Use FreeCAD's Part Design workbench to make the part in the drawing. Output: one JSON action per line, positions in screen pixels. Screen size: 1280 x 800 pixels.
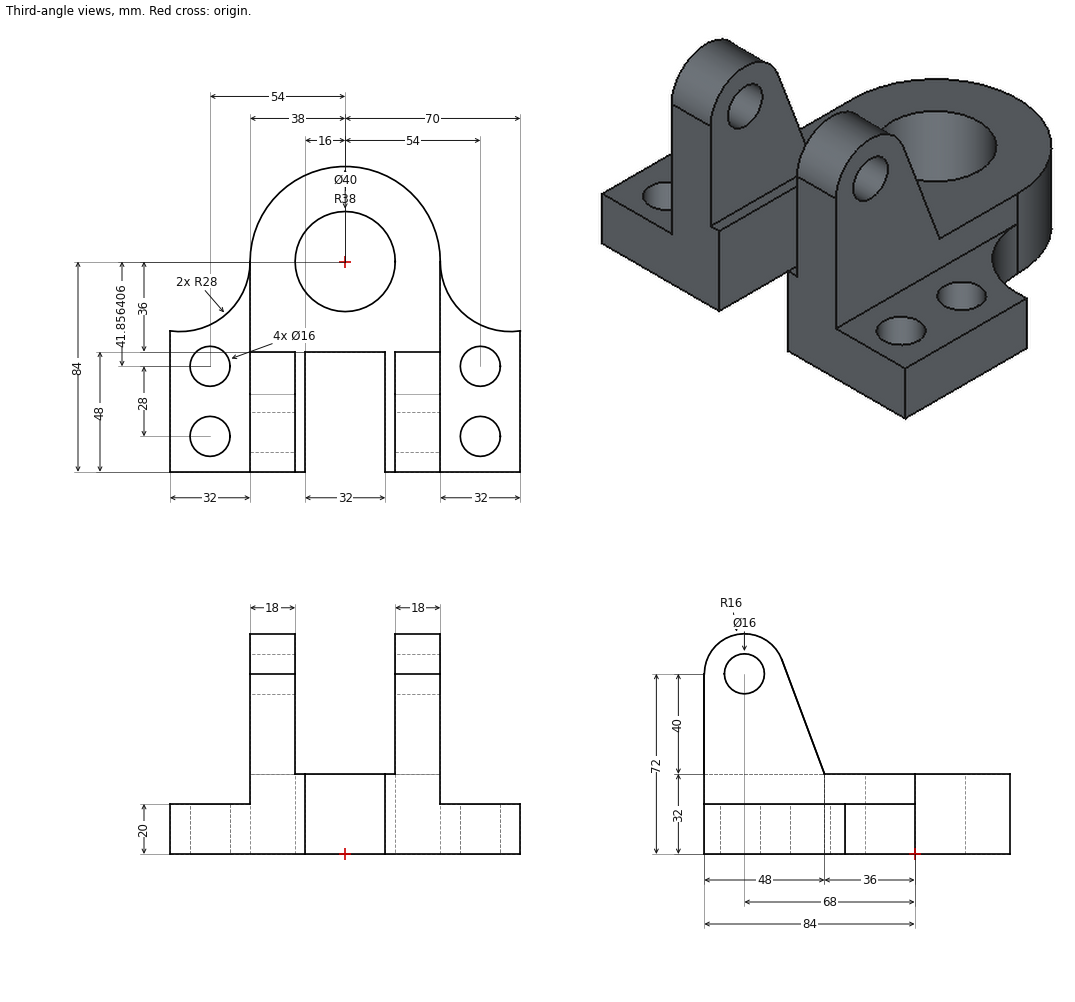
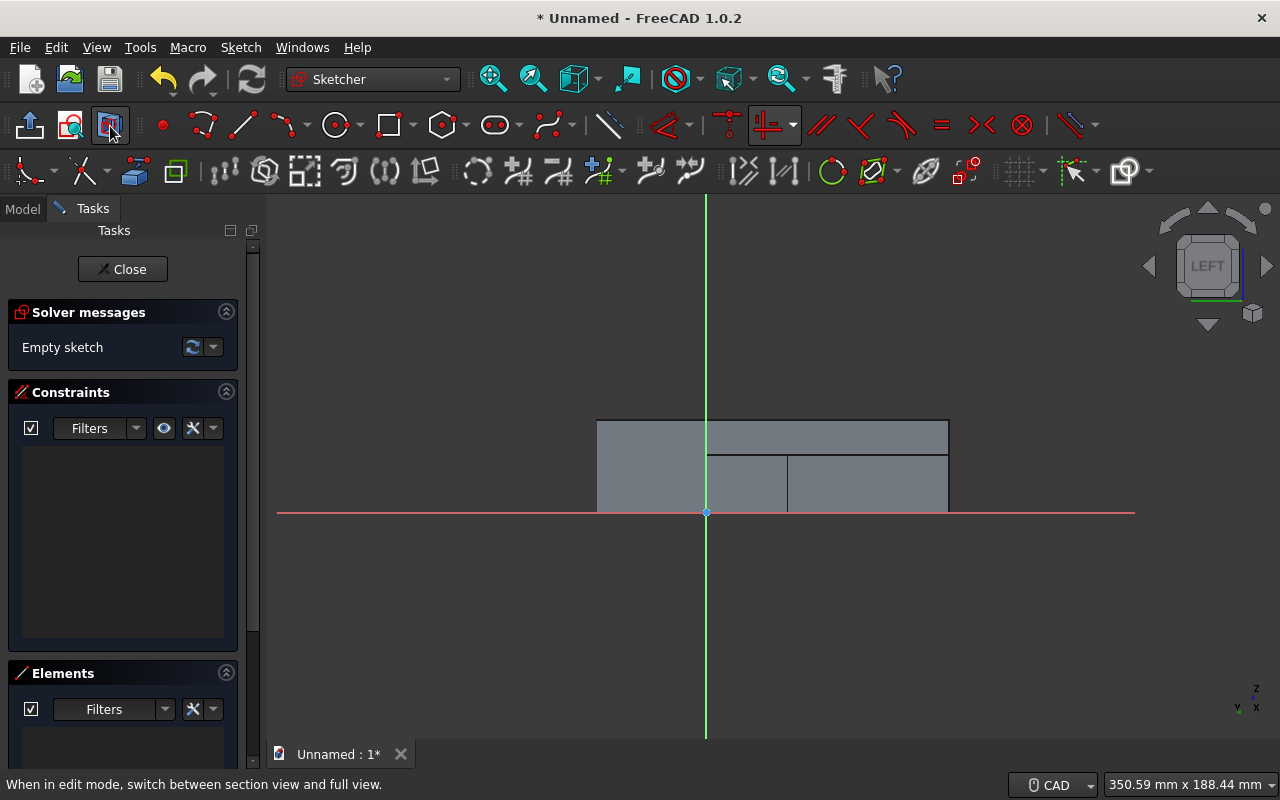
{"action": "scroll", "coordinate": [1079, 222], "scroll_direction": "up", "scroll_amount": 2}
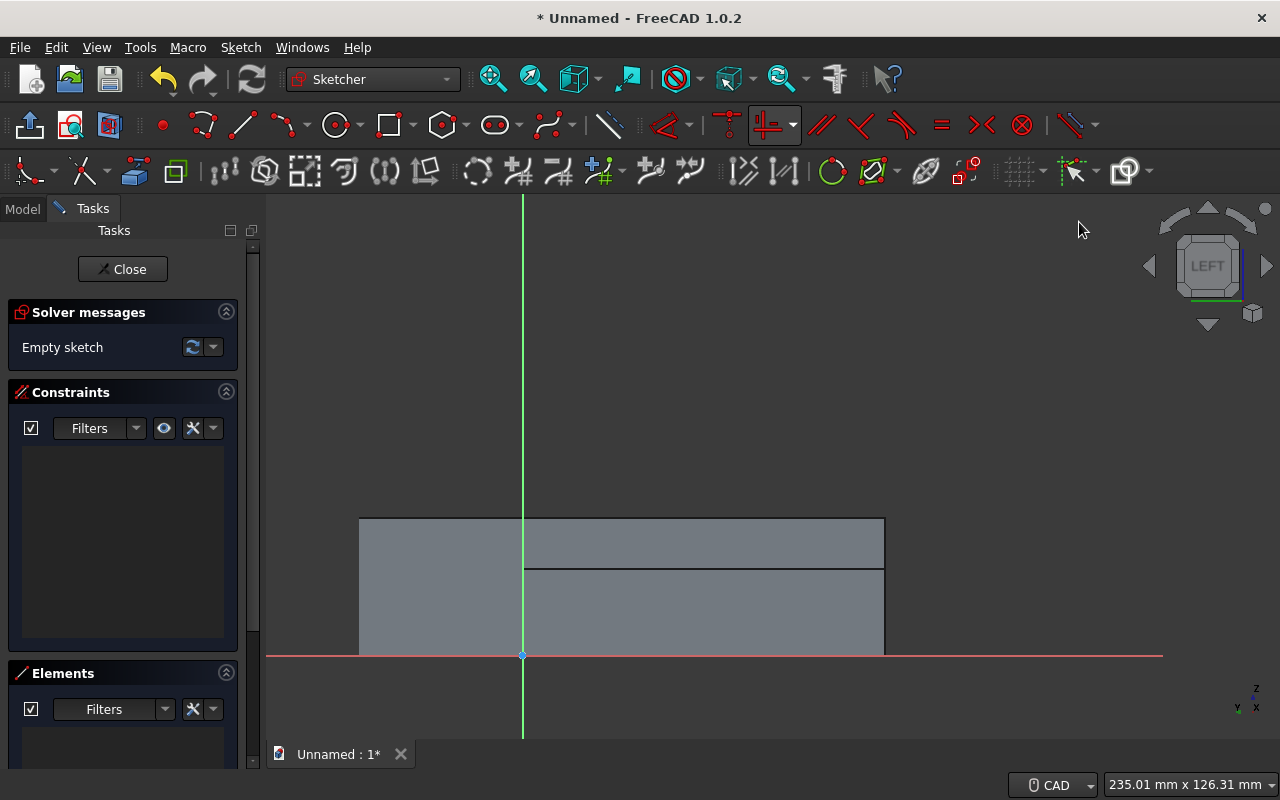
{"action": "left_click", "coordinate": [204, 126]}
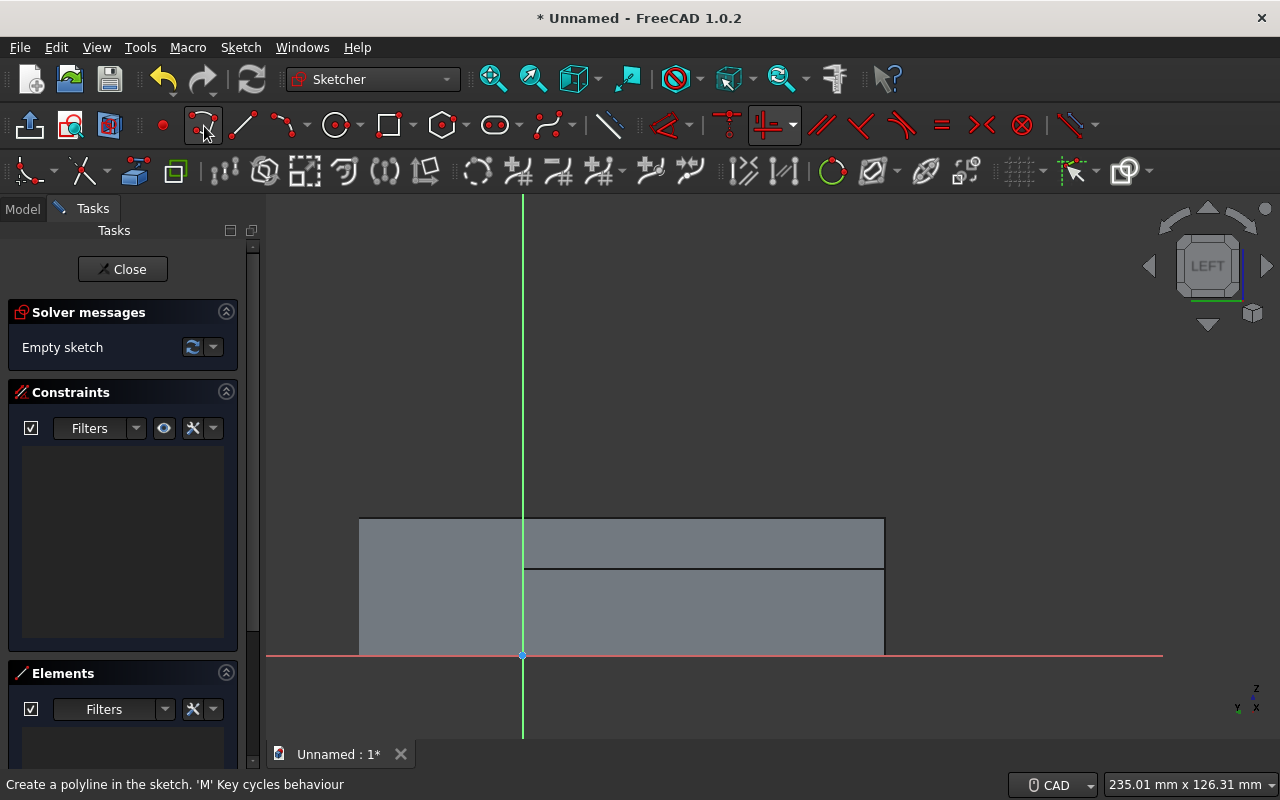
{"action": "left_click", "coordinate": [752, 321]}
{"action": "left_click", "coordinate": [678, 518]}
{"action": "left_click", "coordinate": [885, 518]}
{"action": "left_click", "coordinate": [885, 345]}
{"action": "right_click", "coordinate": [885, 345]}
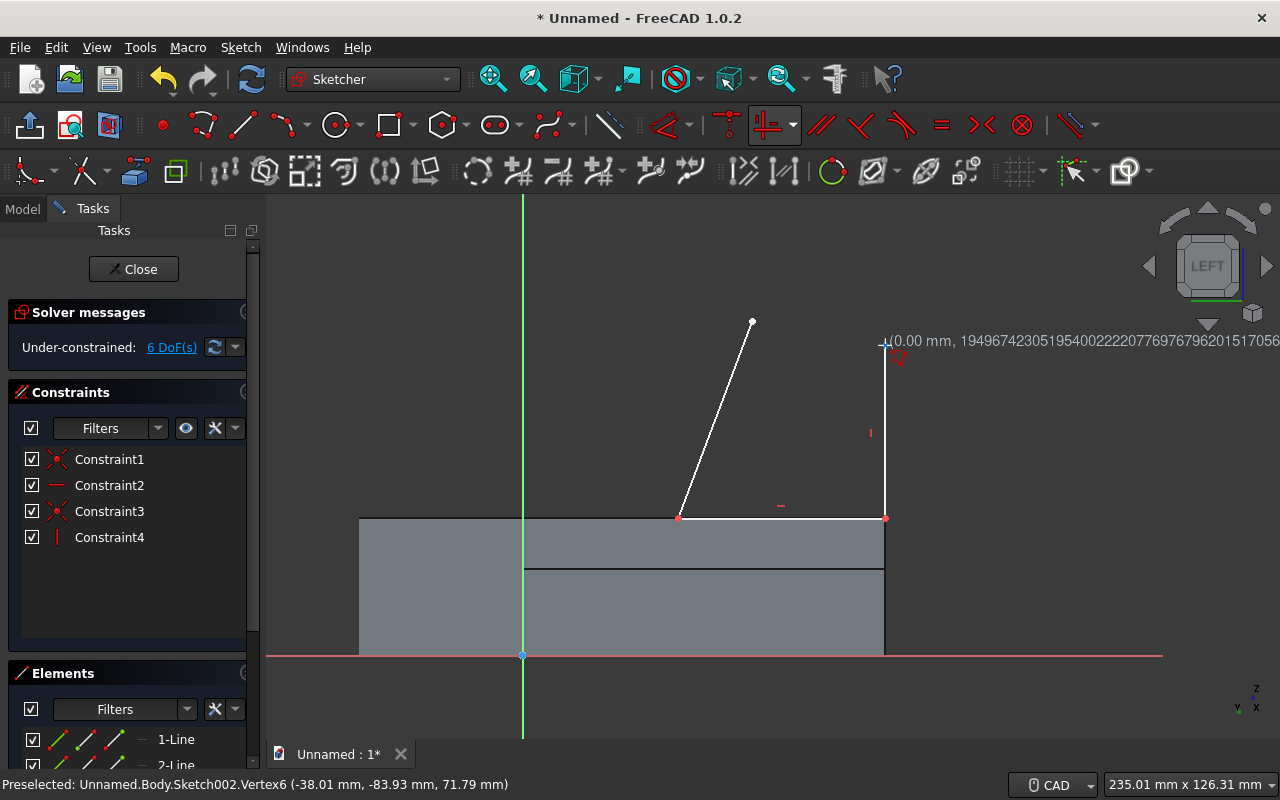
{"action": "left_click", "coordinate": [284, 126]}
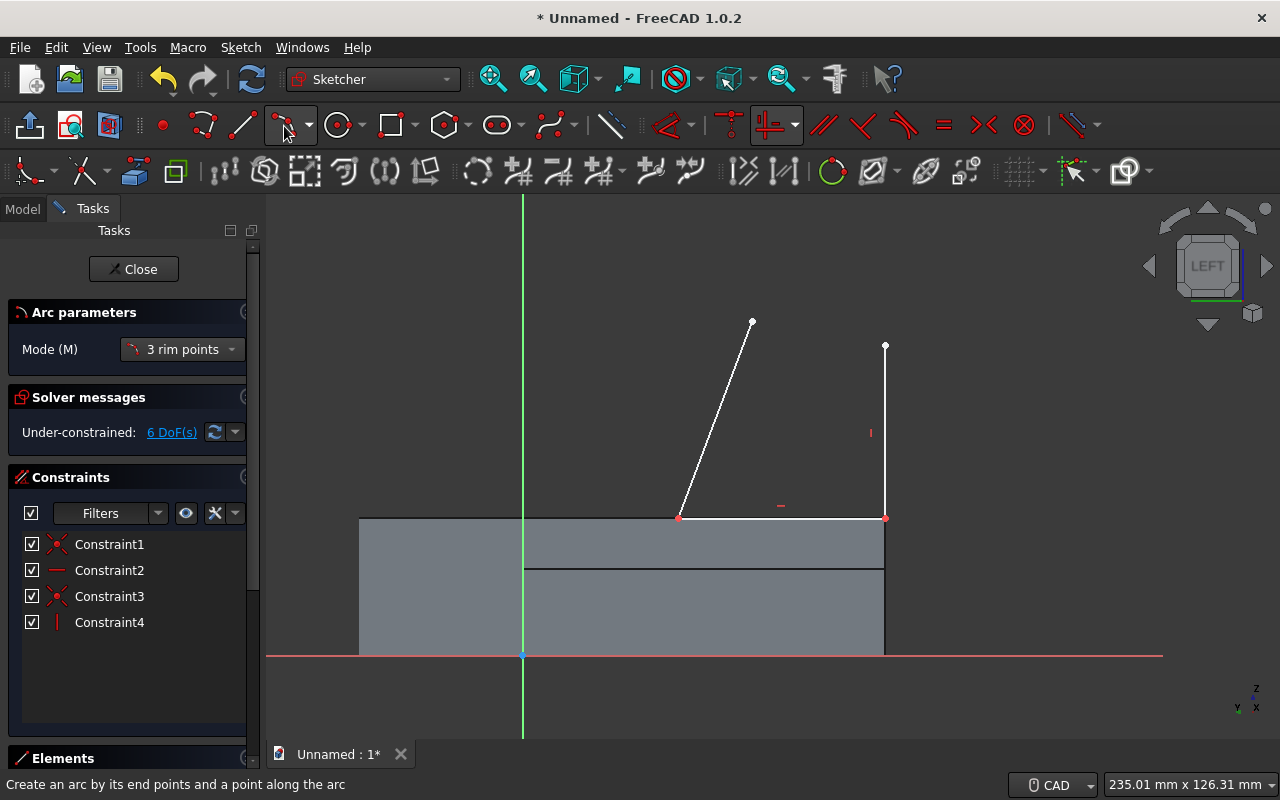
{"action": "left_click", "coordinate": [885, 346]}
{"action": "left_click", "coordinate": [752, 322]}
{"action": "left_click", "coordinate": [829, 277]}
{"action": "key", "text": "Escape"}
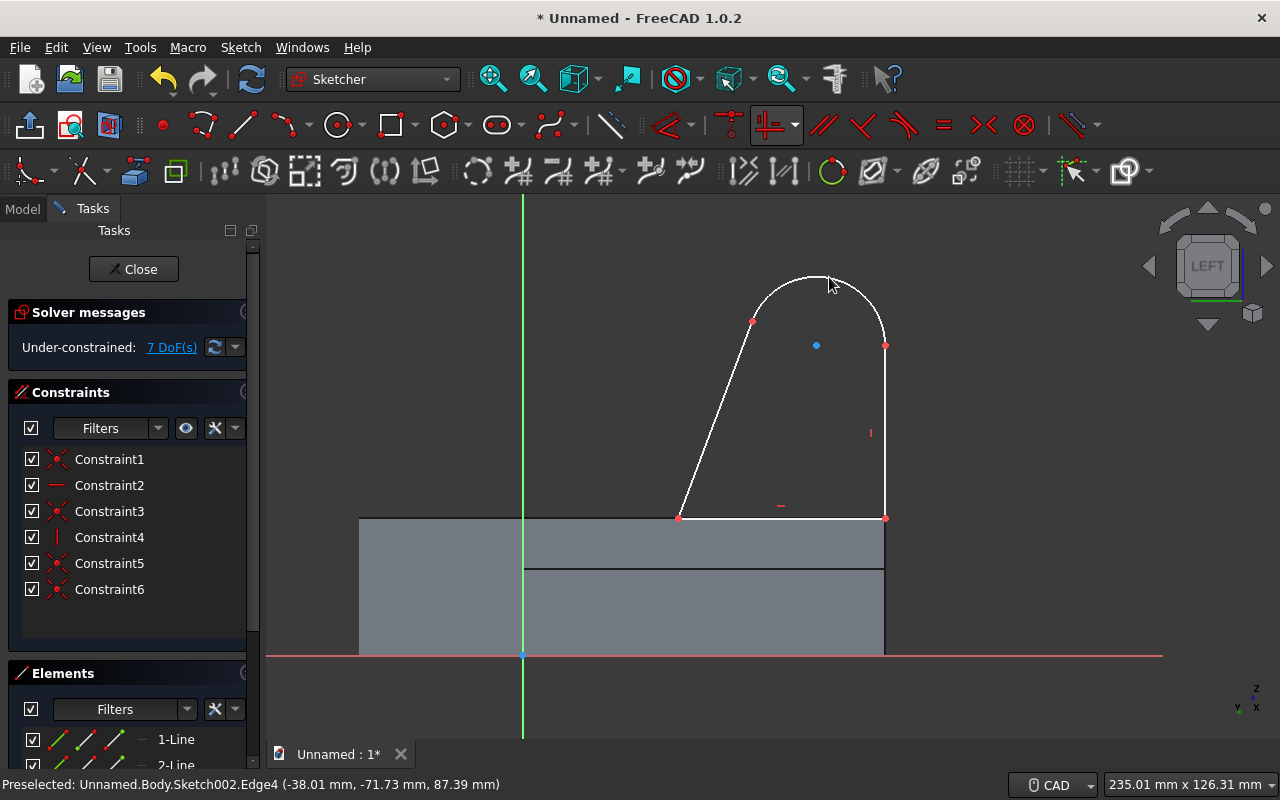
{"action": "left_click", "coordinate": [730, 381]}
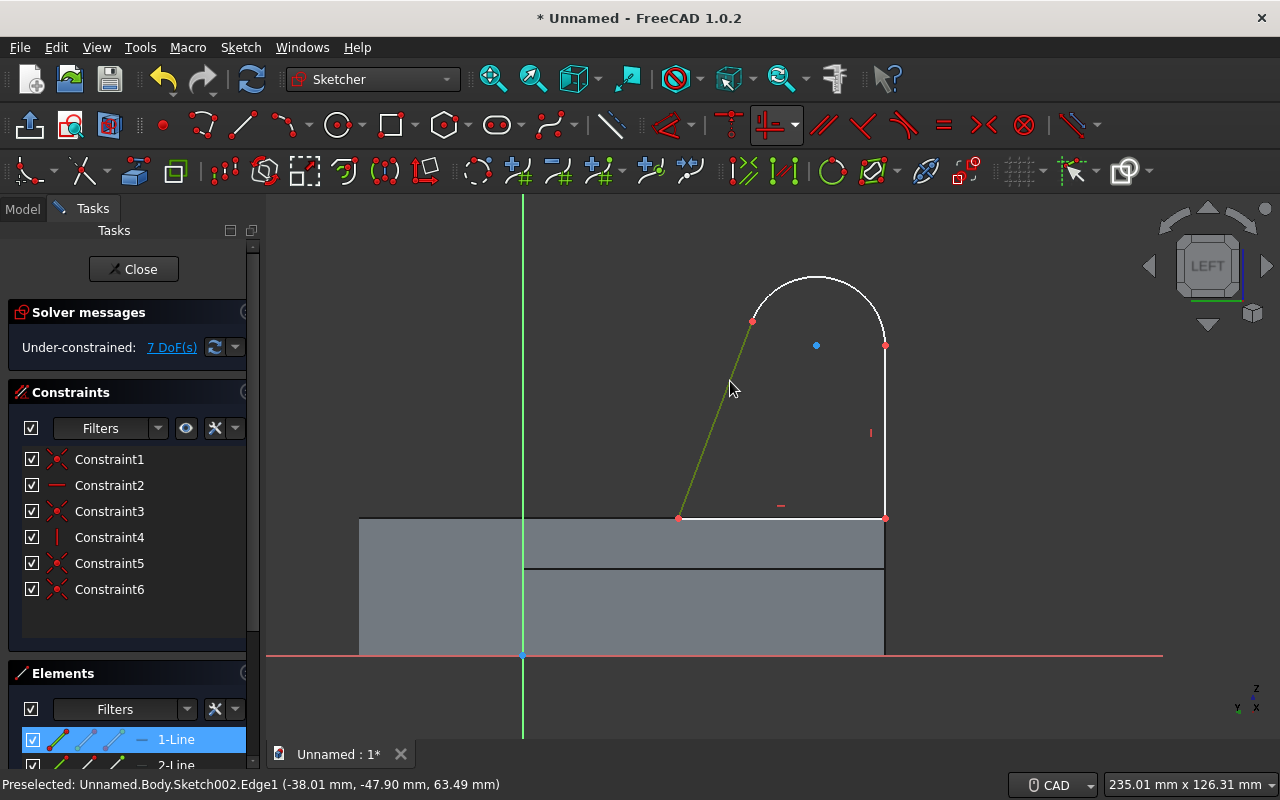
{"action": "left_click", "coordinate": [863, 295]}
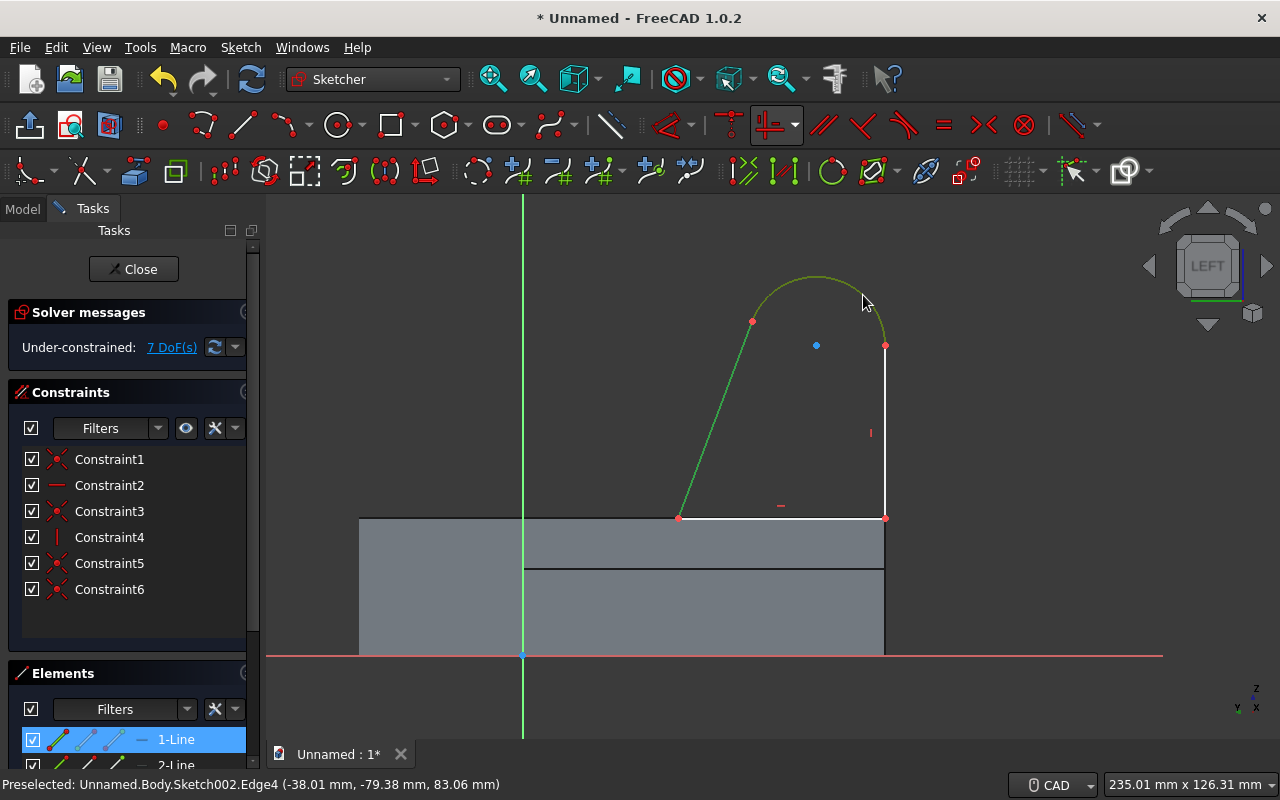
{"action": "left_click", "coordinate": [904, 126]}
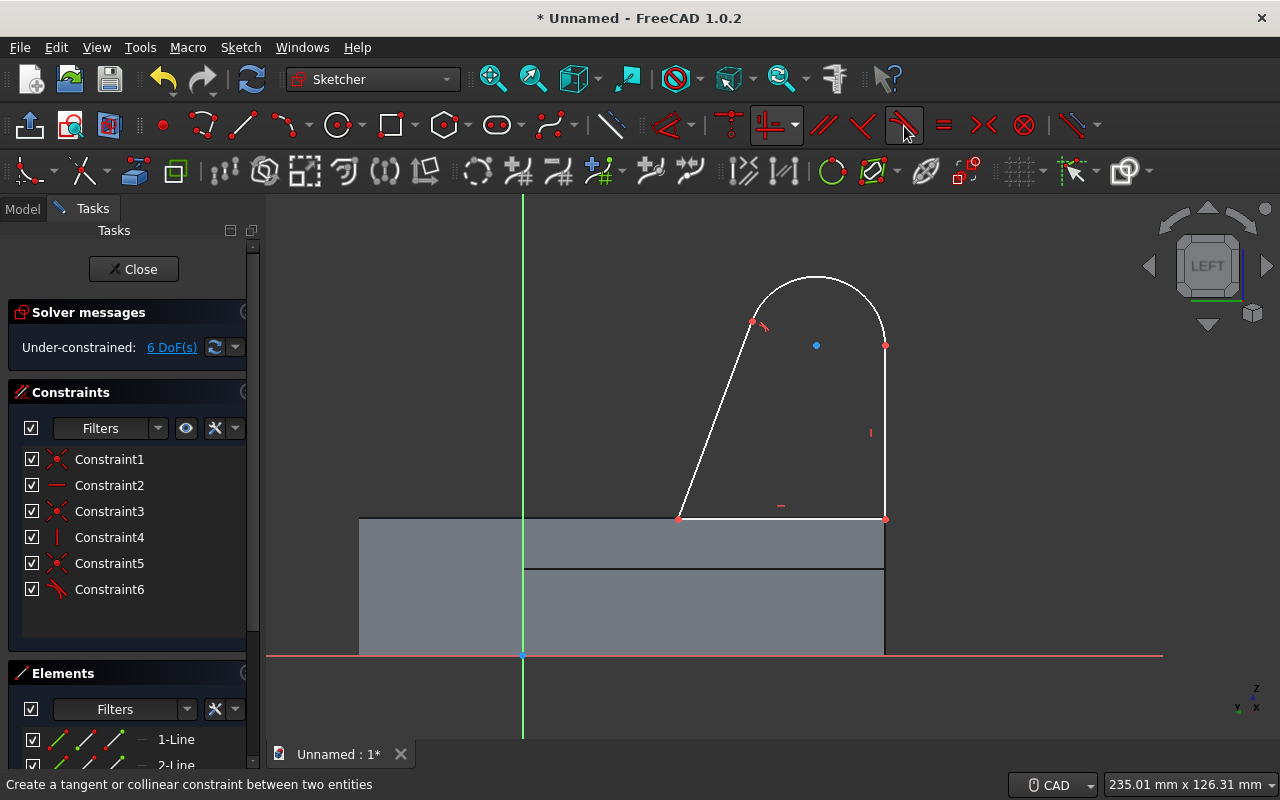
{"action": "left_click", "coordinate": [885, 467]}